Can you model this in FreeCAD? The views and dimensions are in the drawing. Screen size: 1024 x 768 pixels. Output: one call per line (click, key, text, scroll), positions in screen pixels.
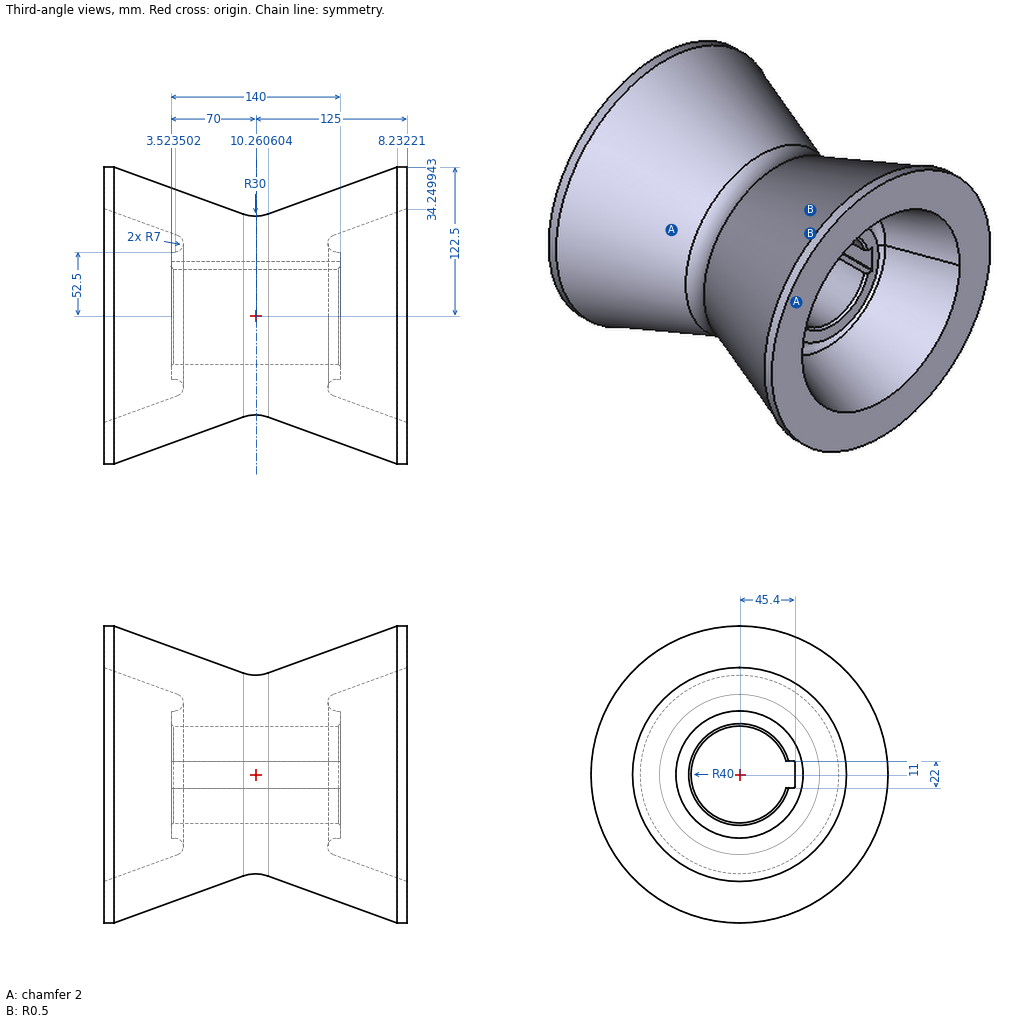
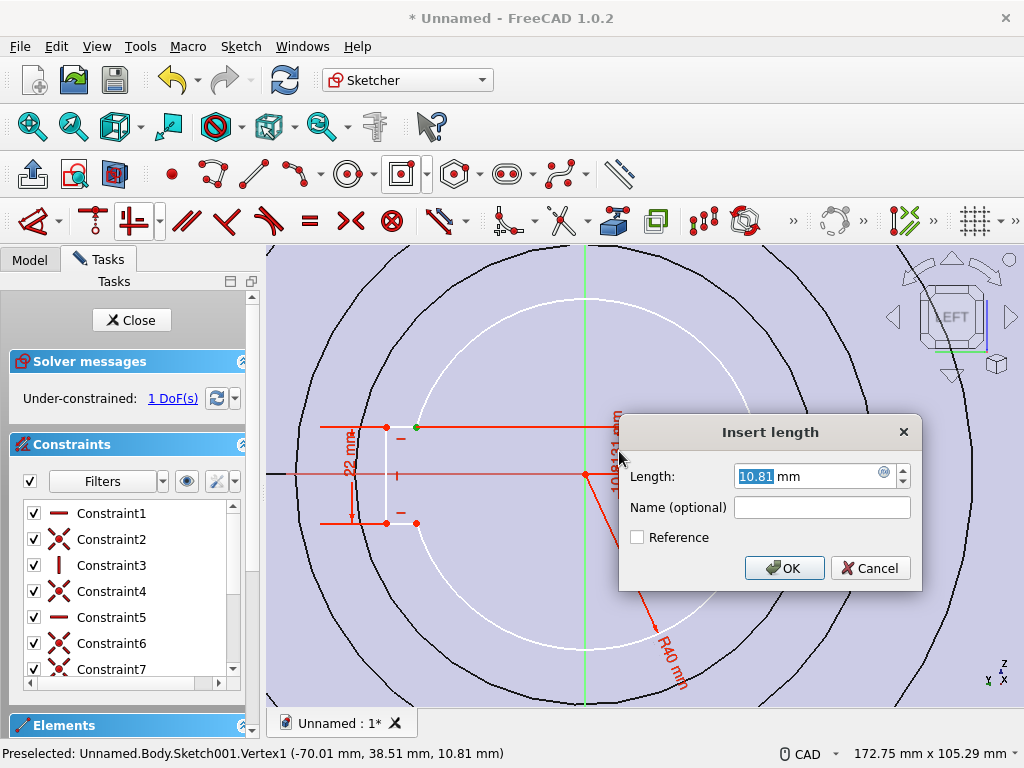
text(11)
key(Return)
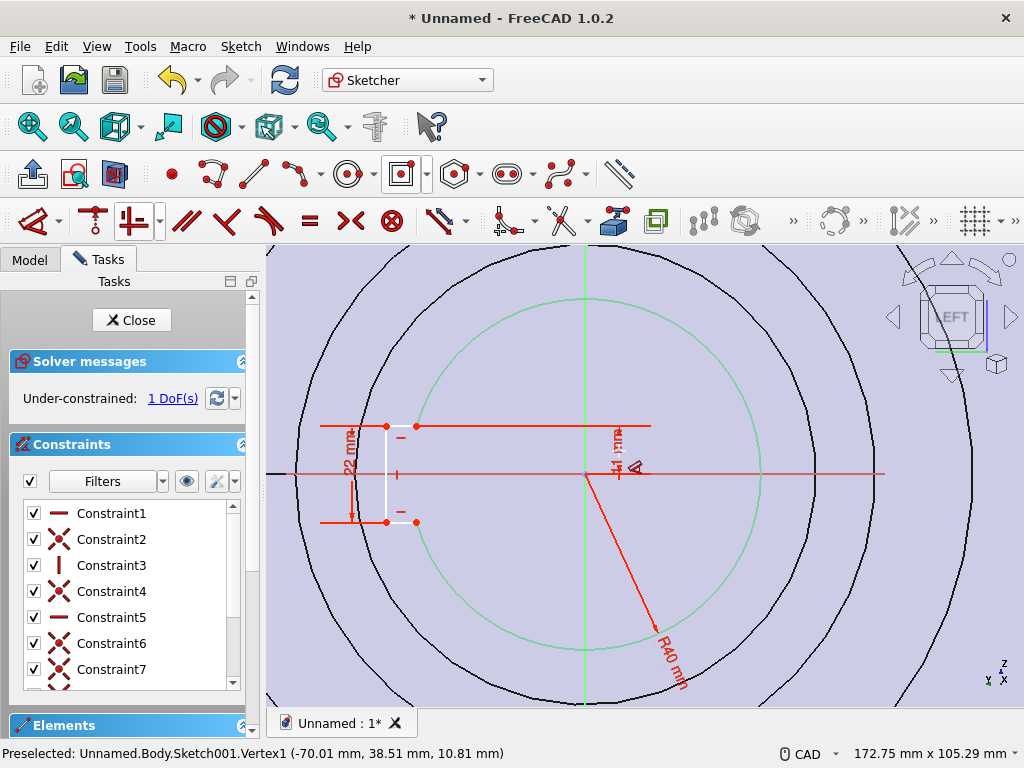
click(386, 426)
click(486, 392)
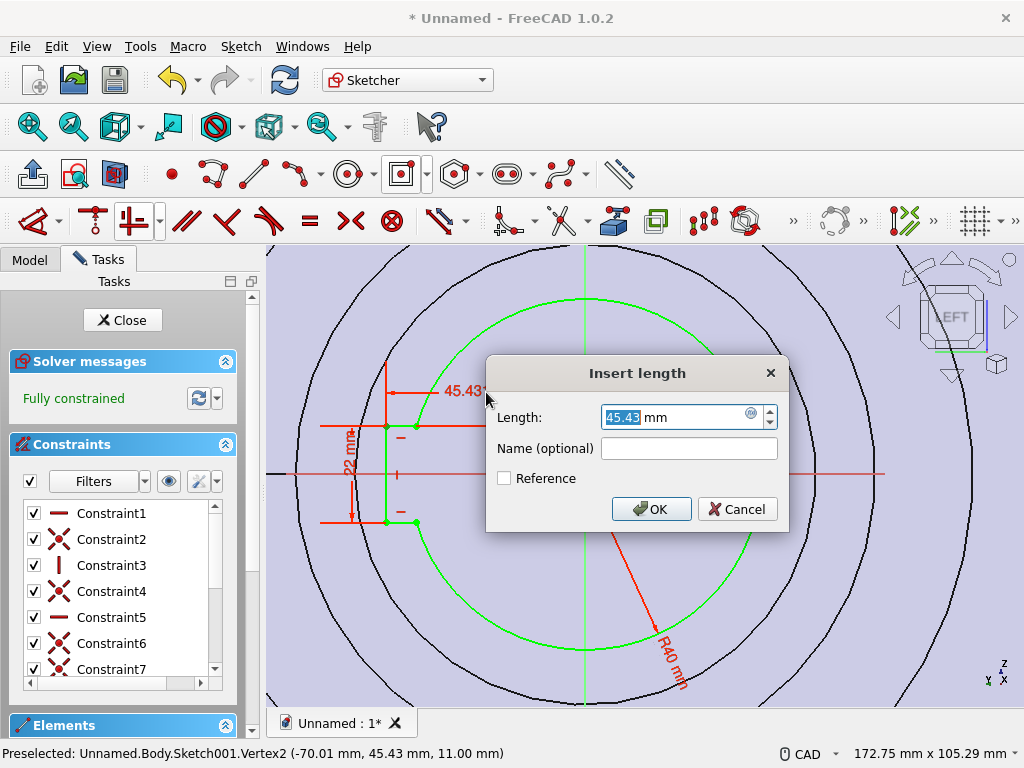
text(45.4)
key(Return)
key(Escape)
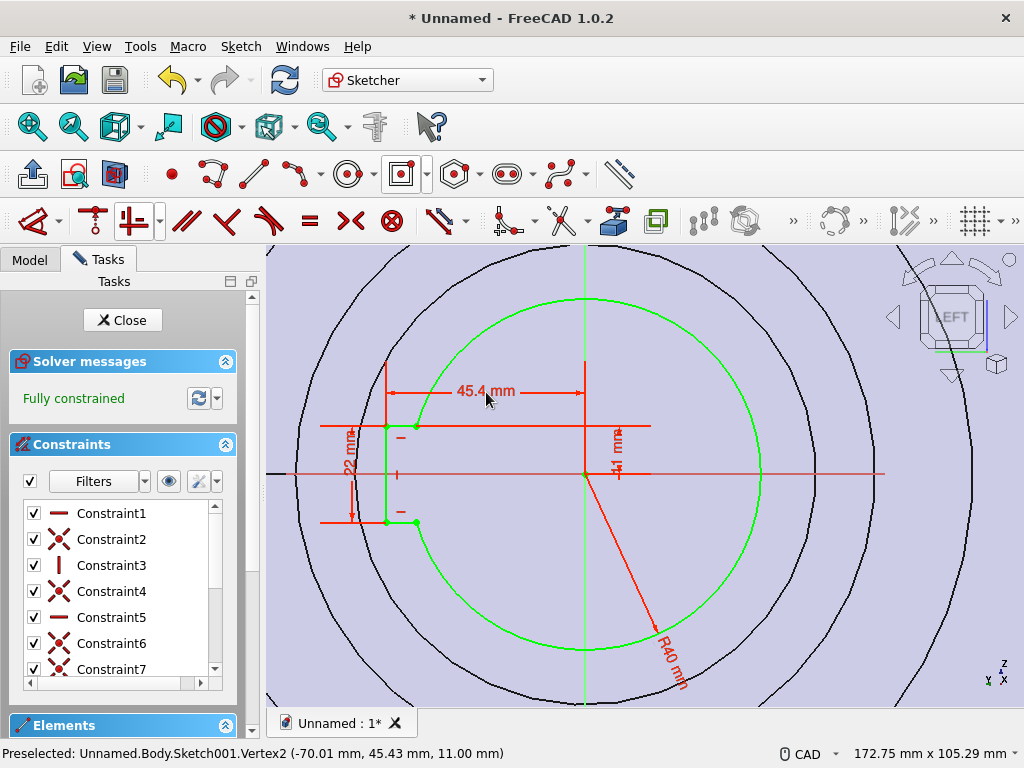
click(123, 320)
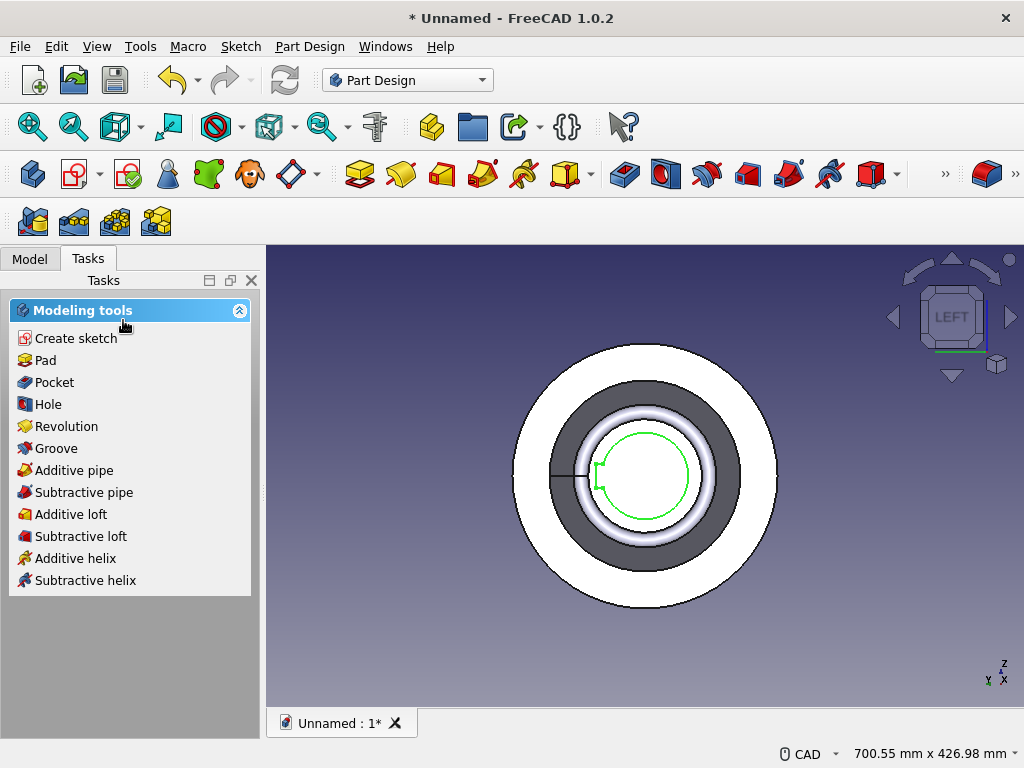
click(625, 174)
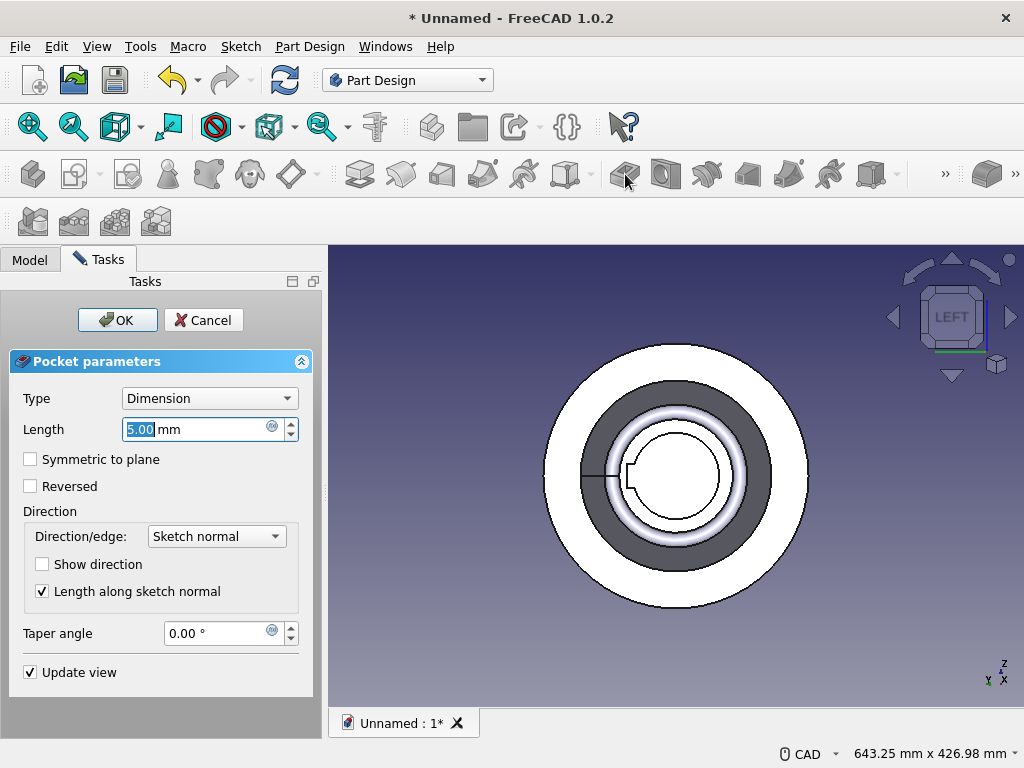
click(210, 398)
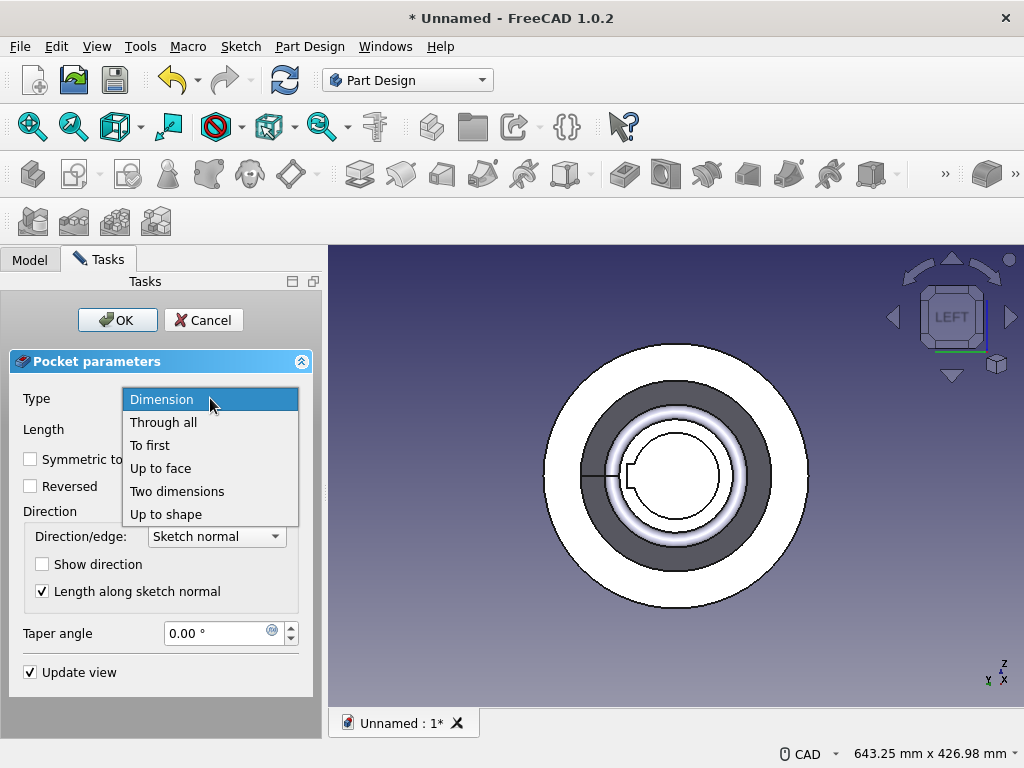
click(208, 422)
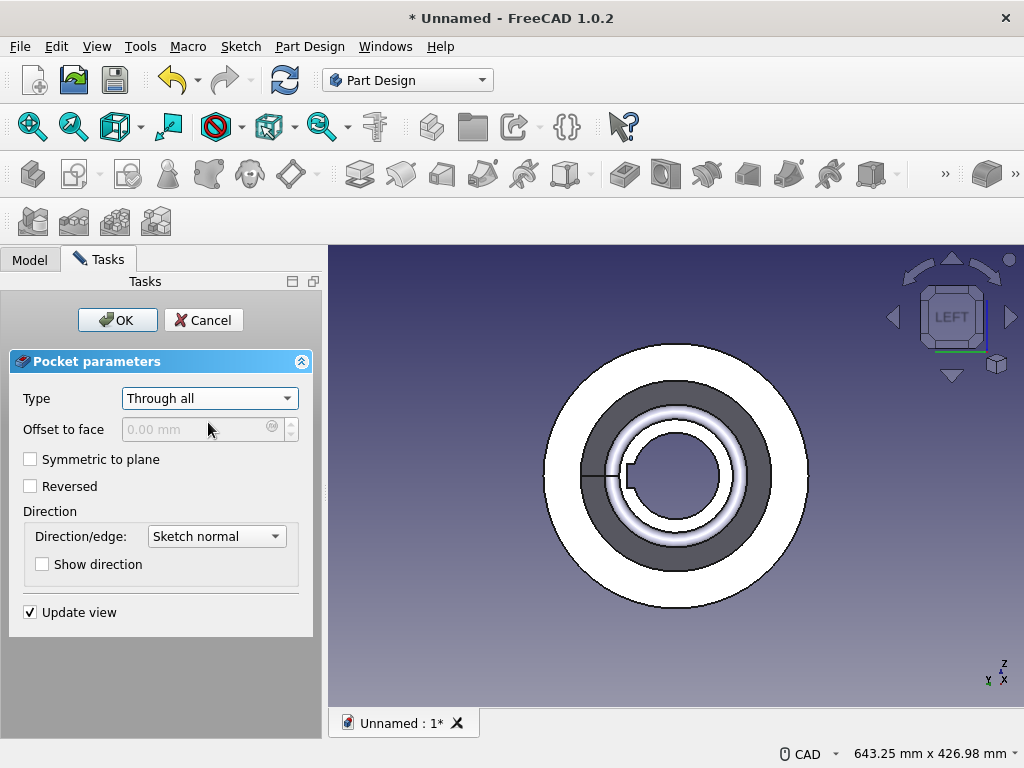
click(118, 320)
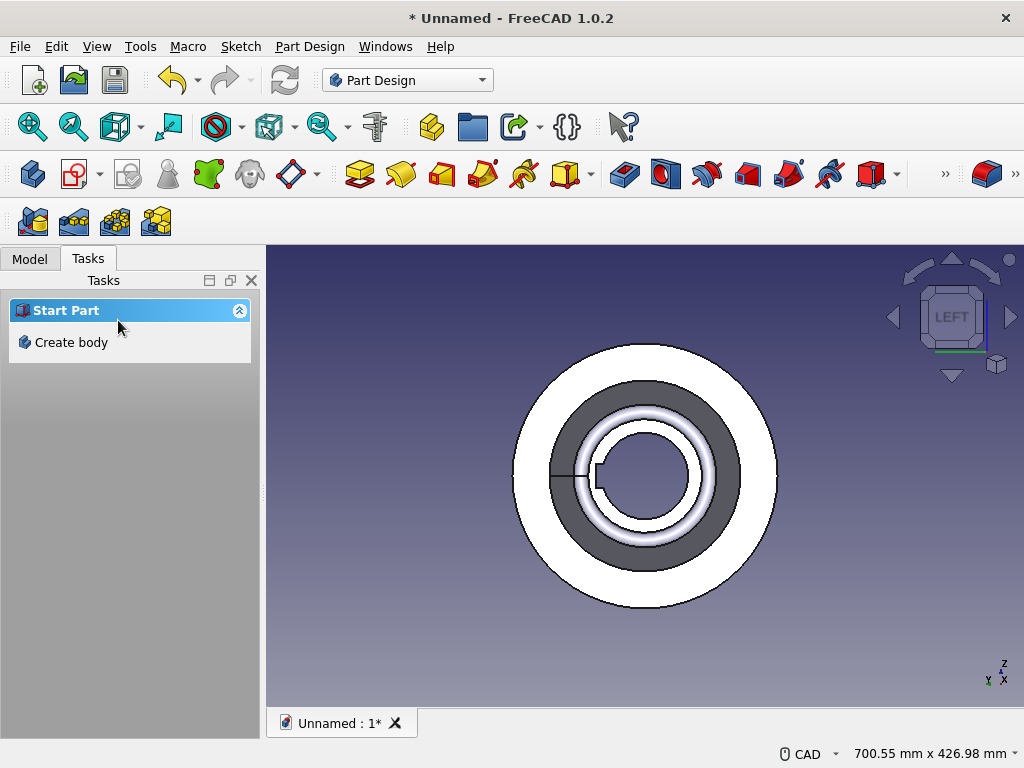
click(688, 475)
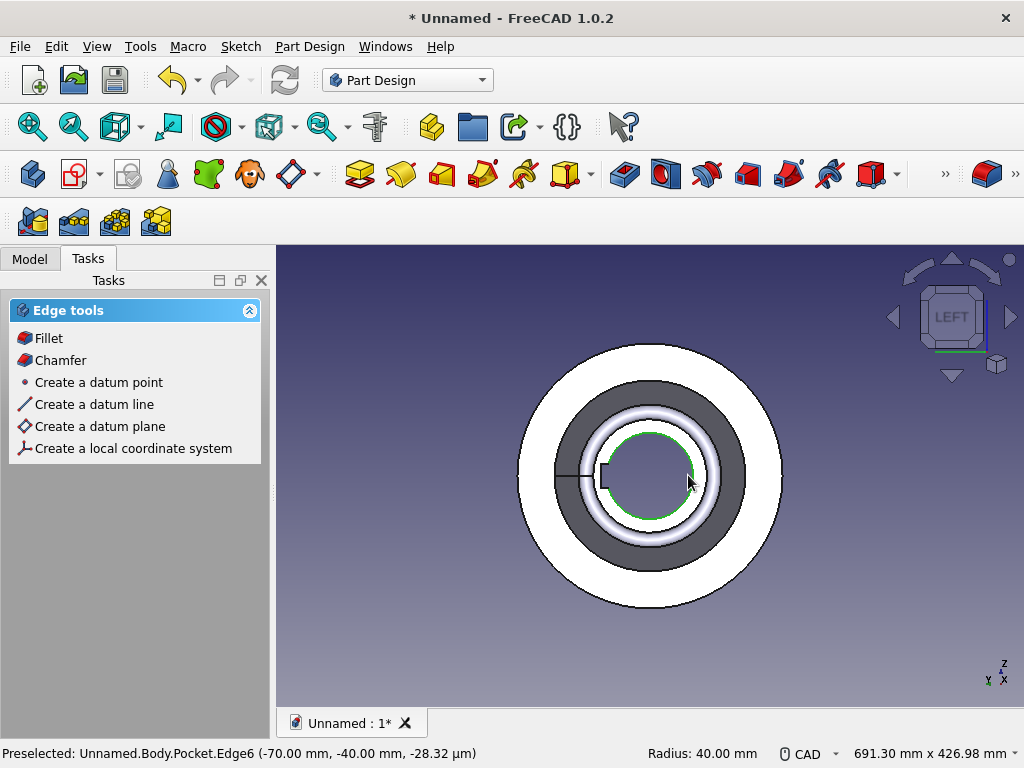
key(0)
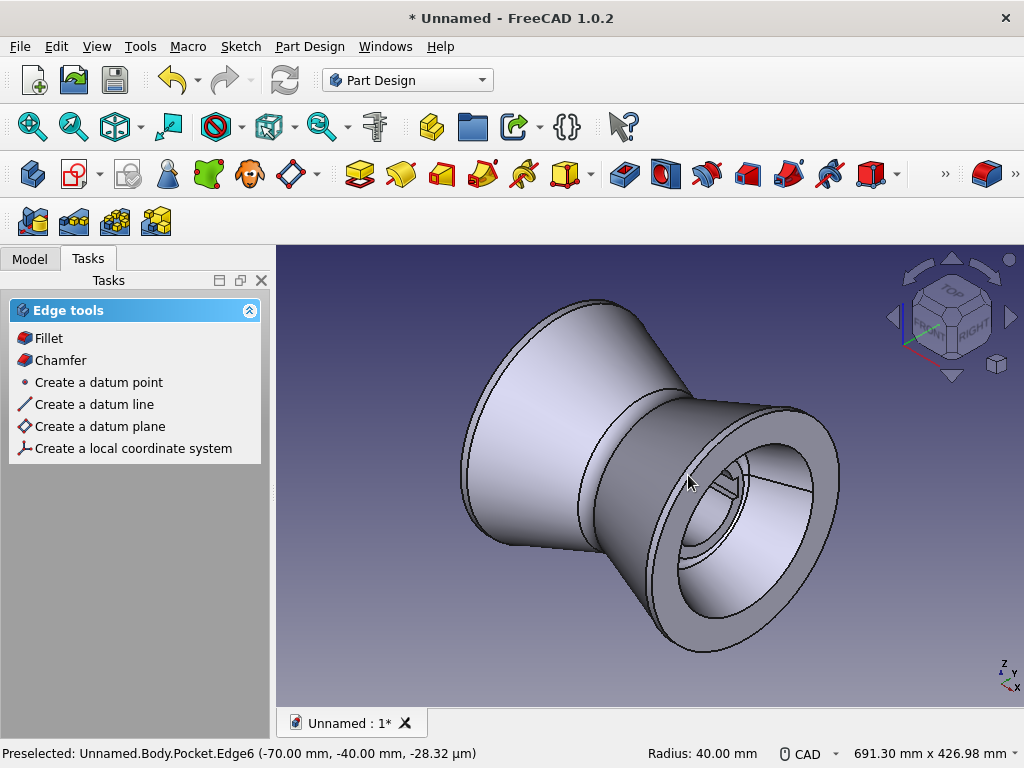
click(691, 545, ctrl)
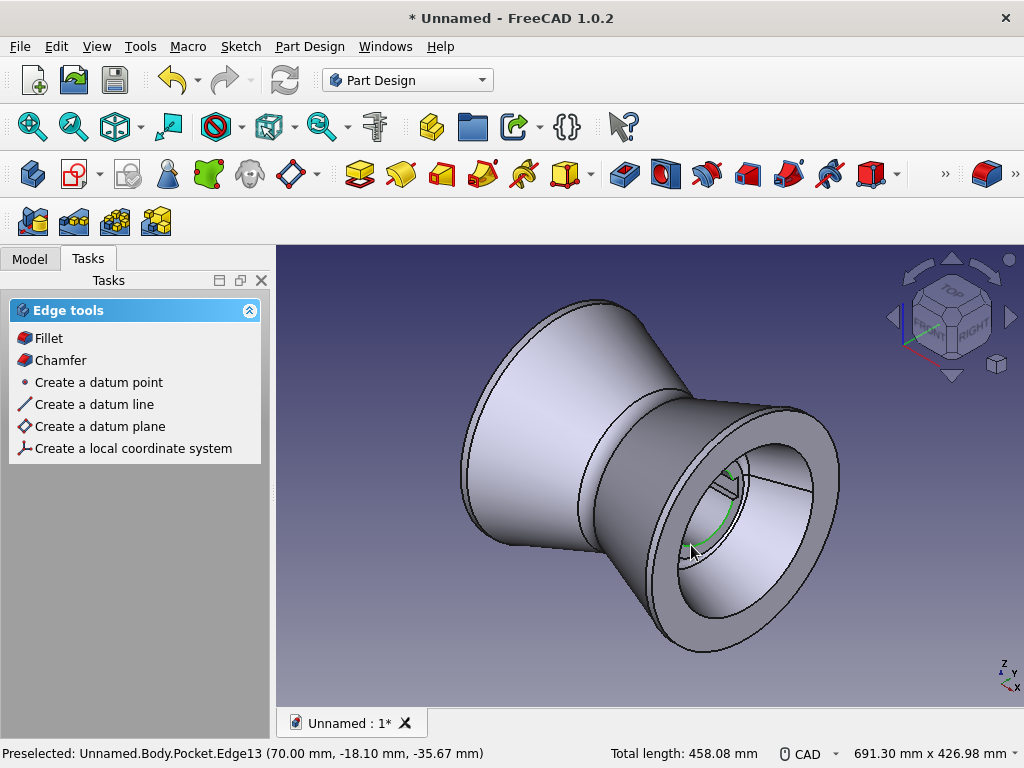
click(135, 360)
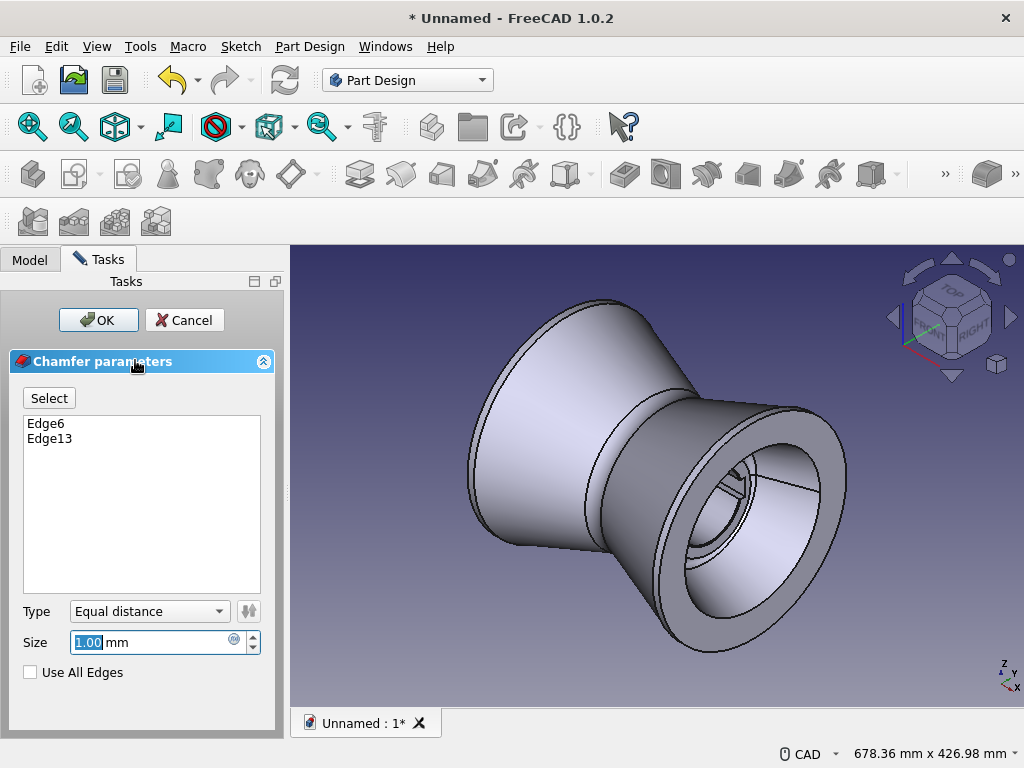
text(2)
key(Tab)